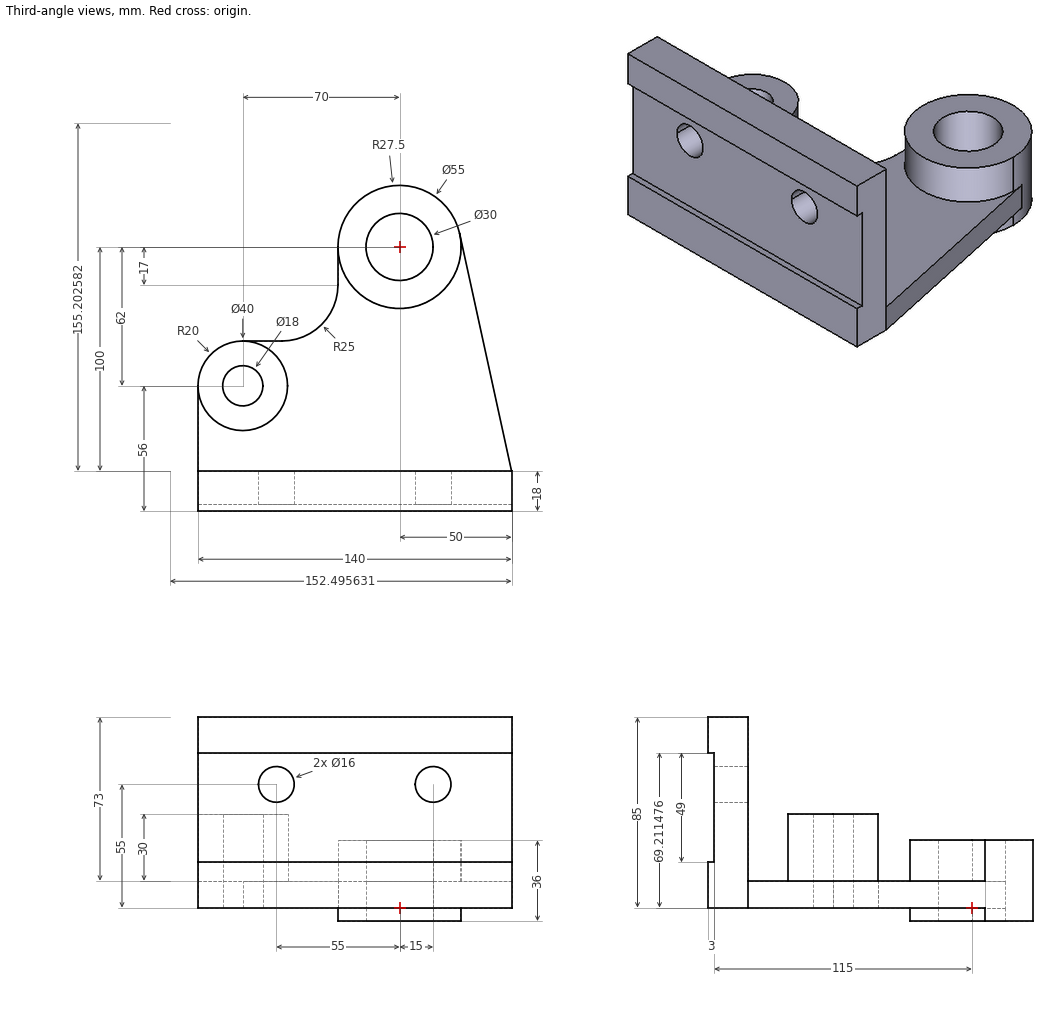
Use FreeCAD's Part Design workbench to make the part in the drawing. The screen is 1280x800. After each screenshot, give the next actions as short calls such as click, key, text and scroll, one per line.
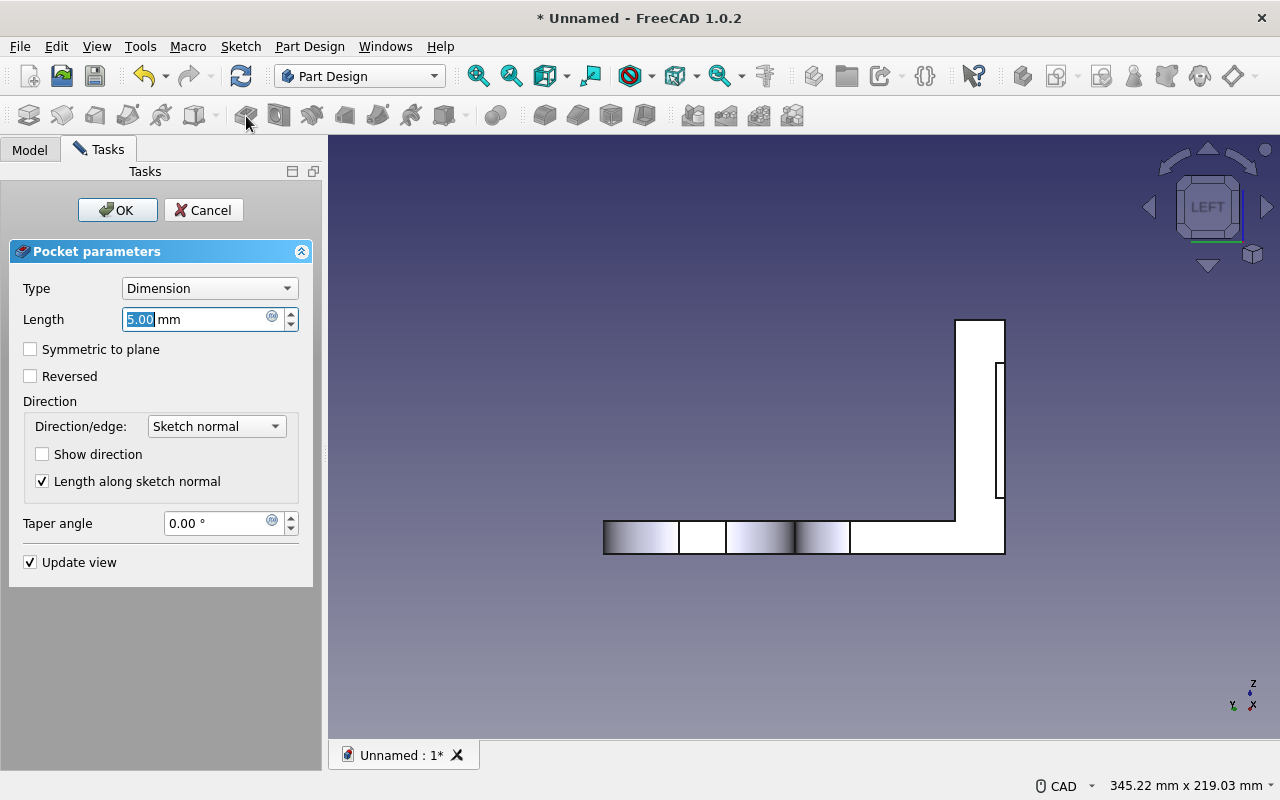
click(210, 288)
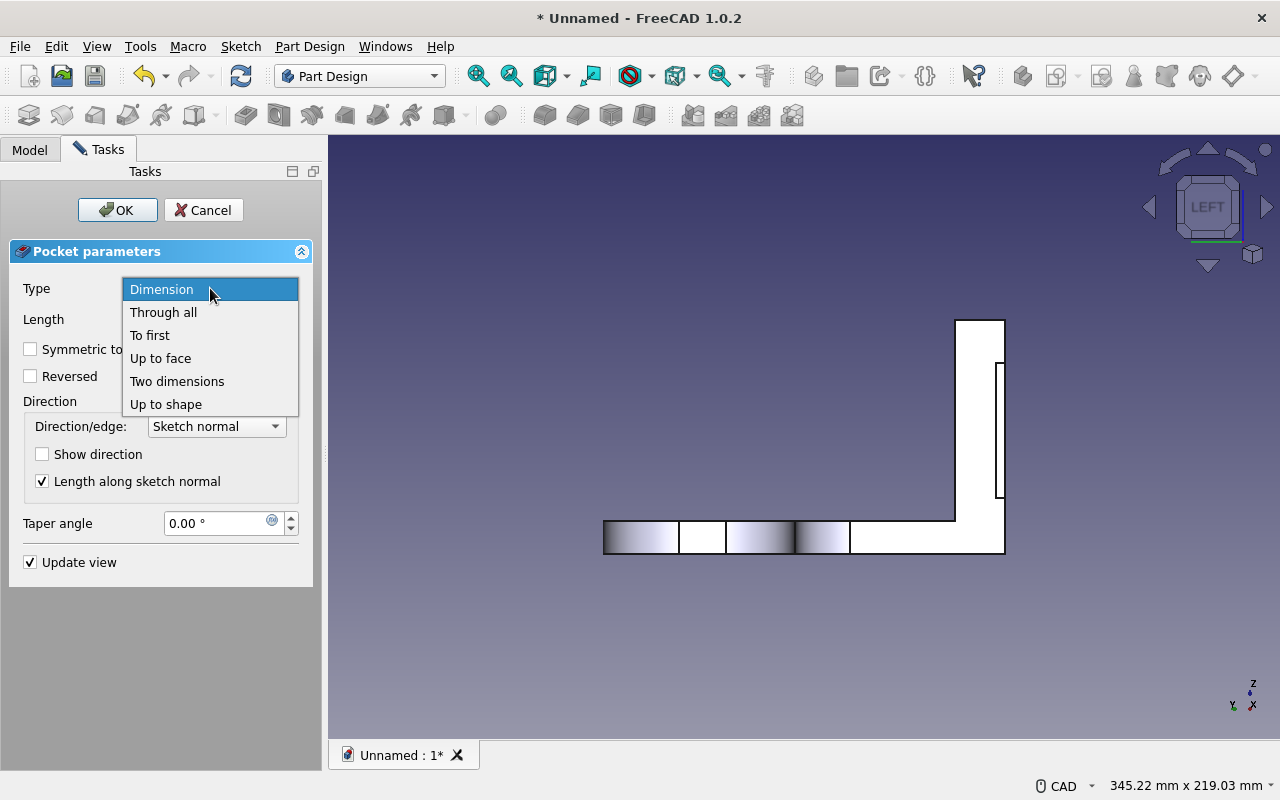
click(208, 312)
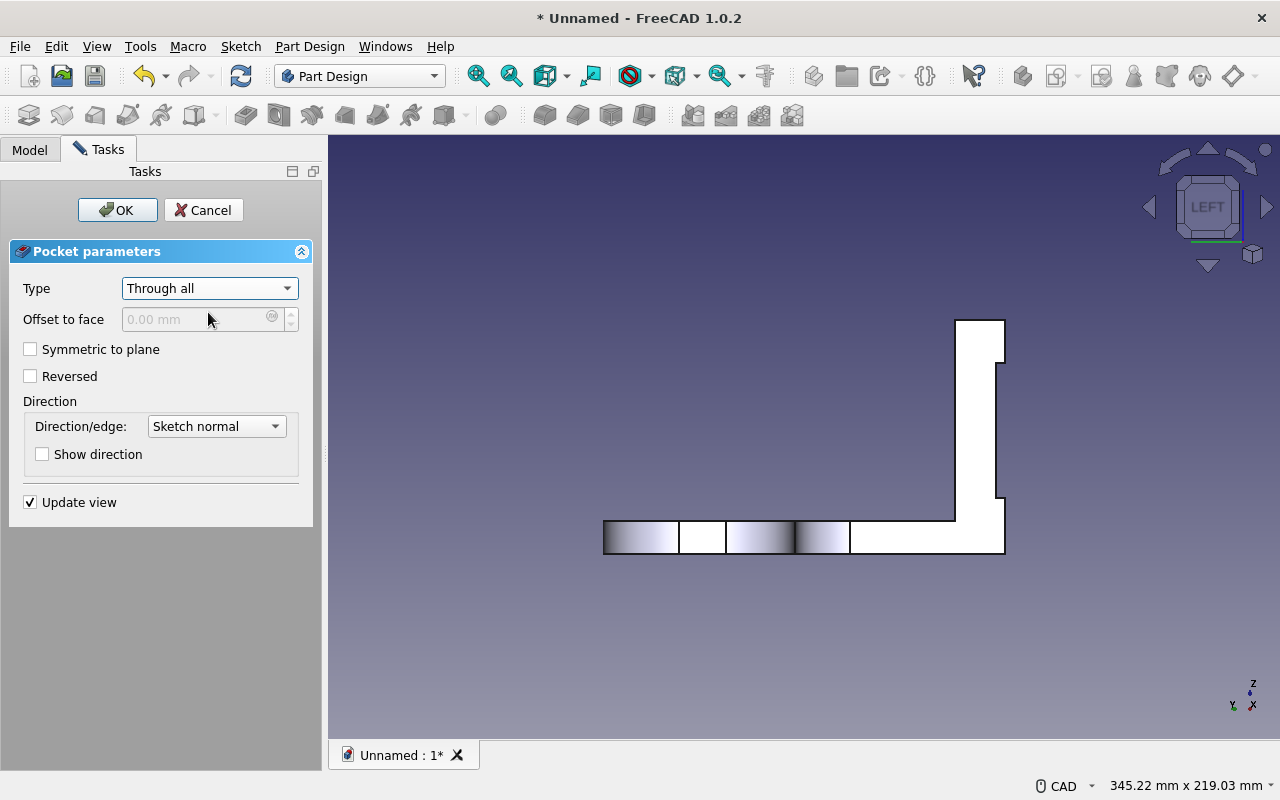
click(118, 210)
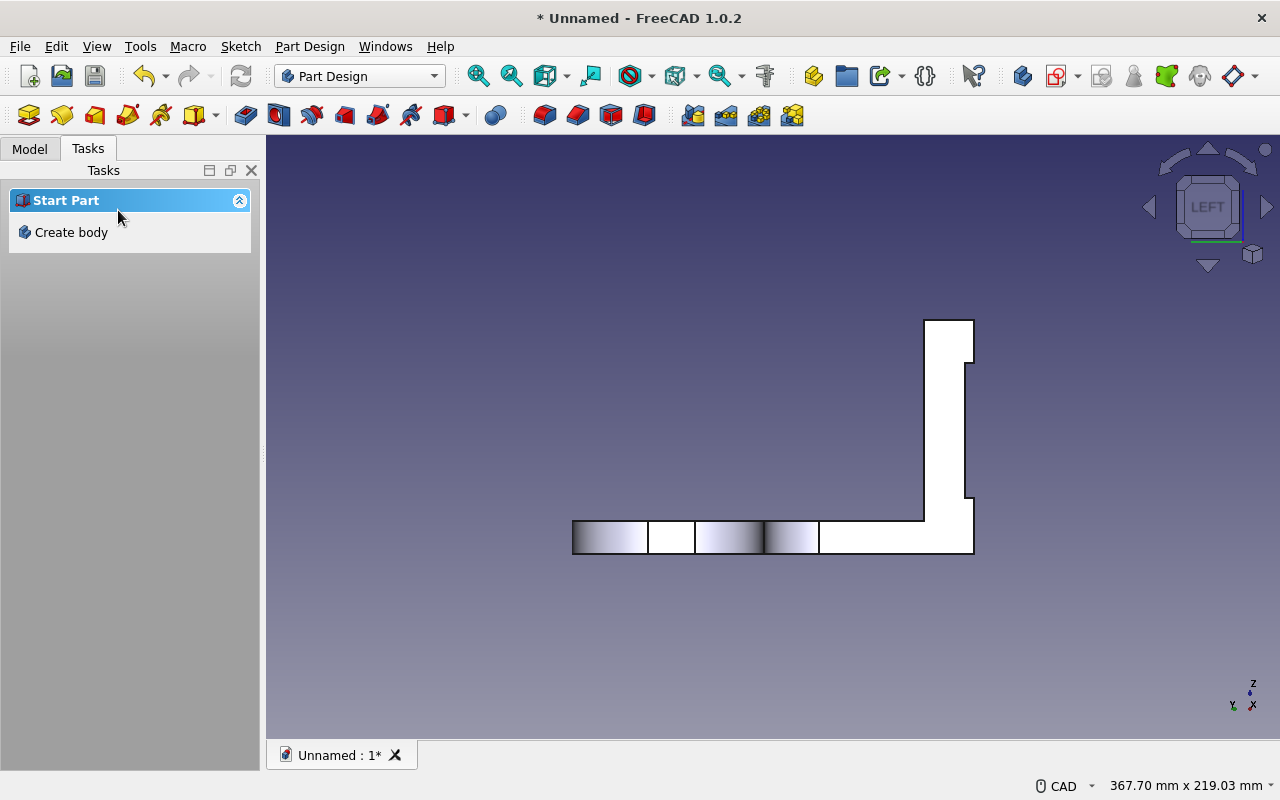
click(479, 76)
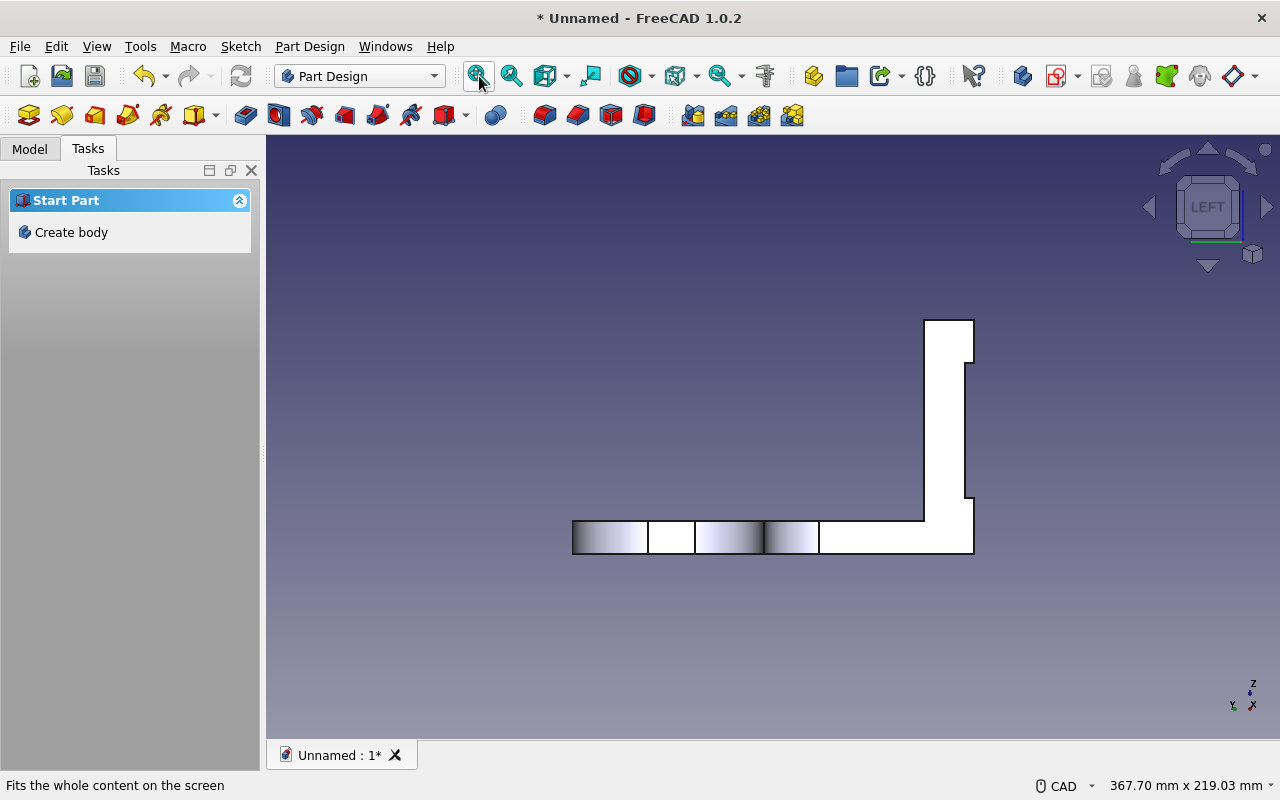
key(0)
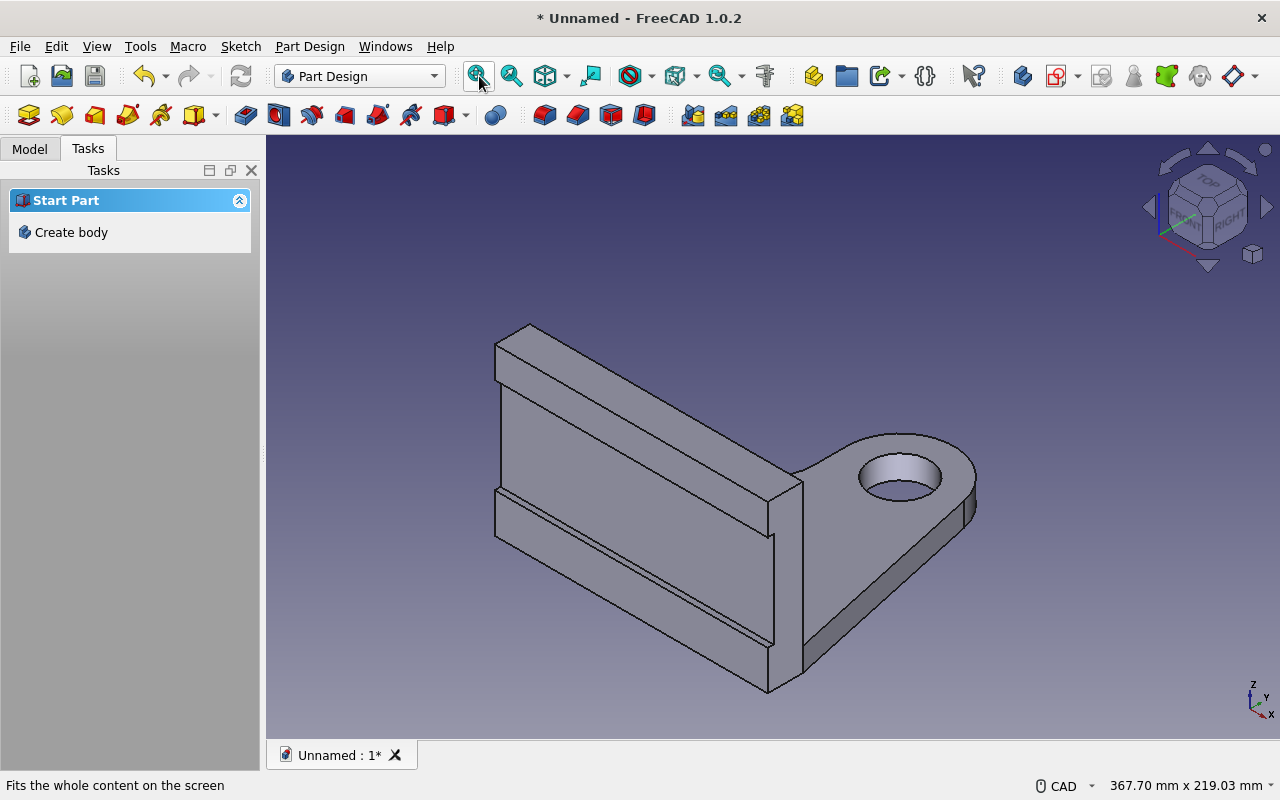
click(830, 517)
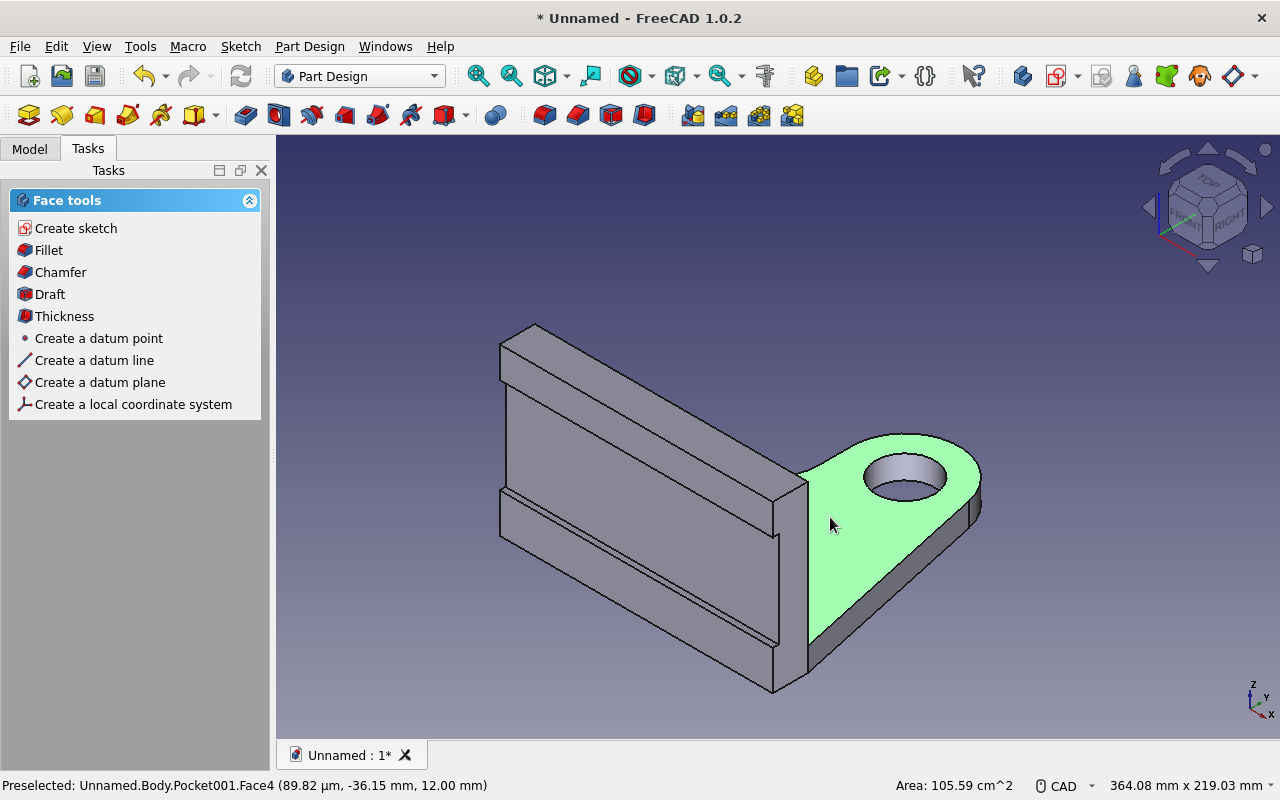
click(1056, 76)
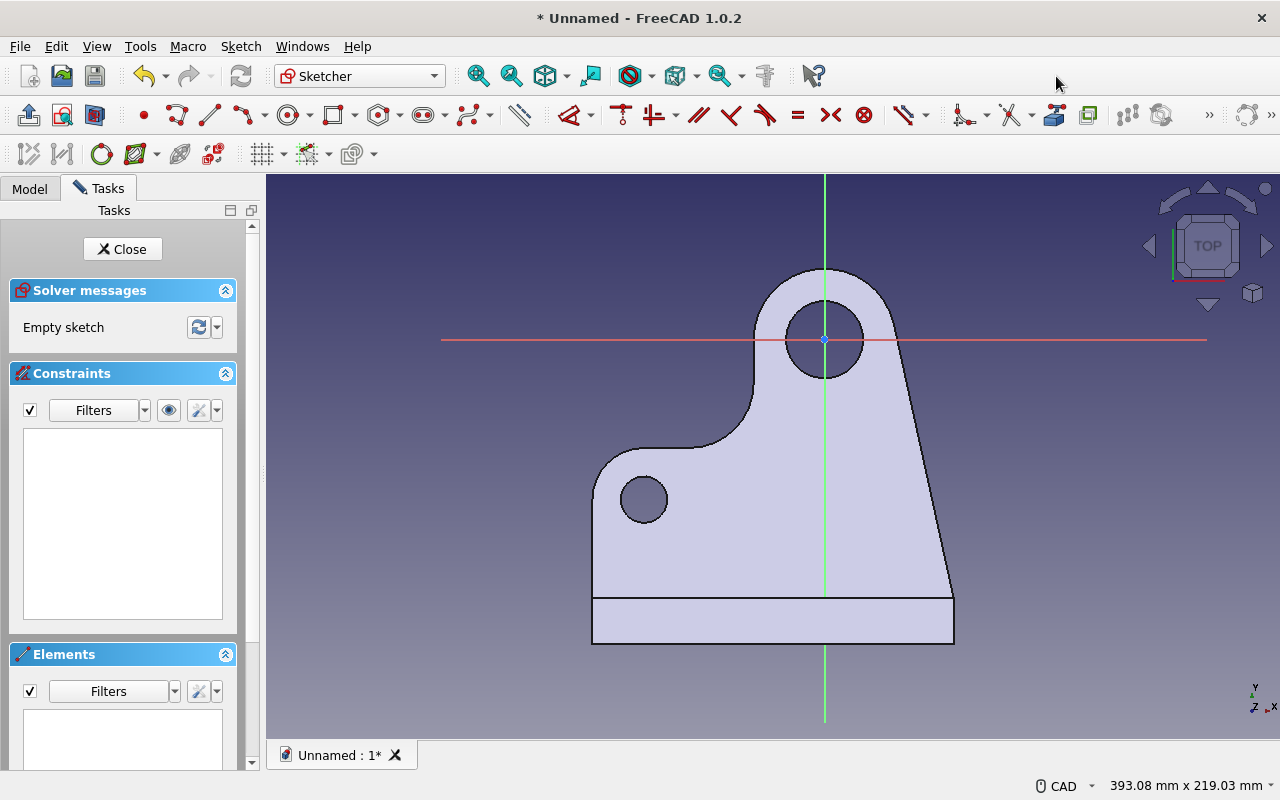
click(95, 116)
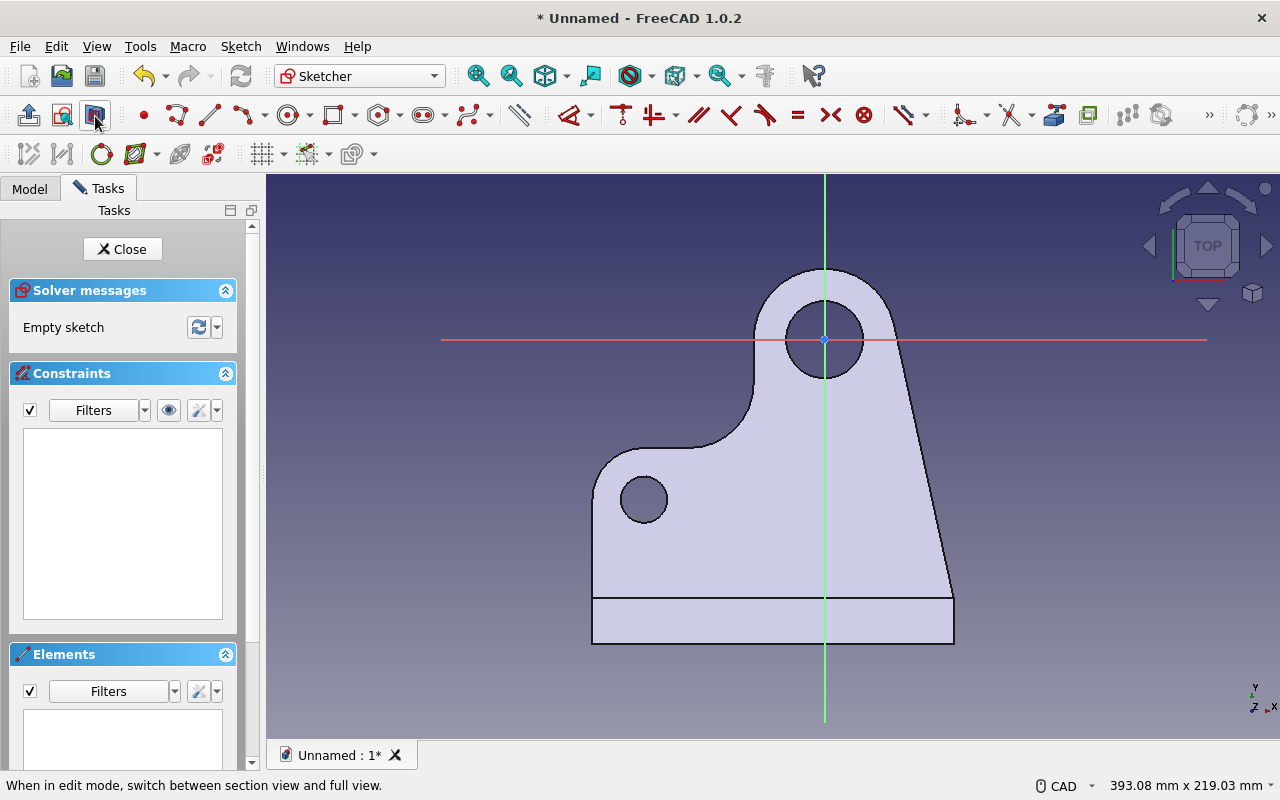
scroll(894, 272, up, 5)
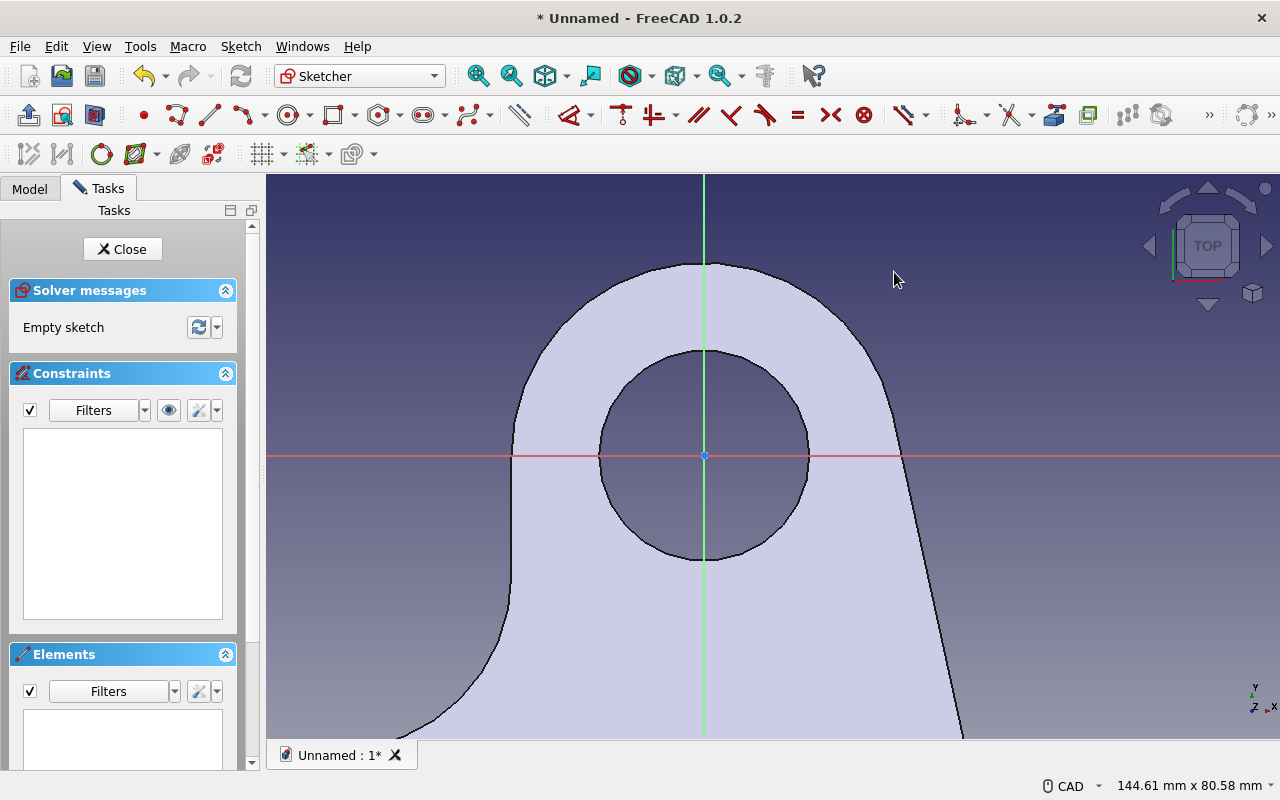
key(g)
key(c)